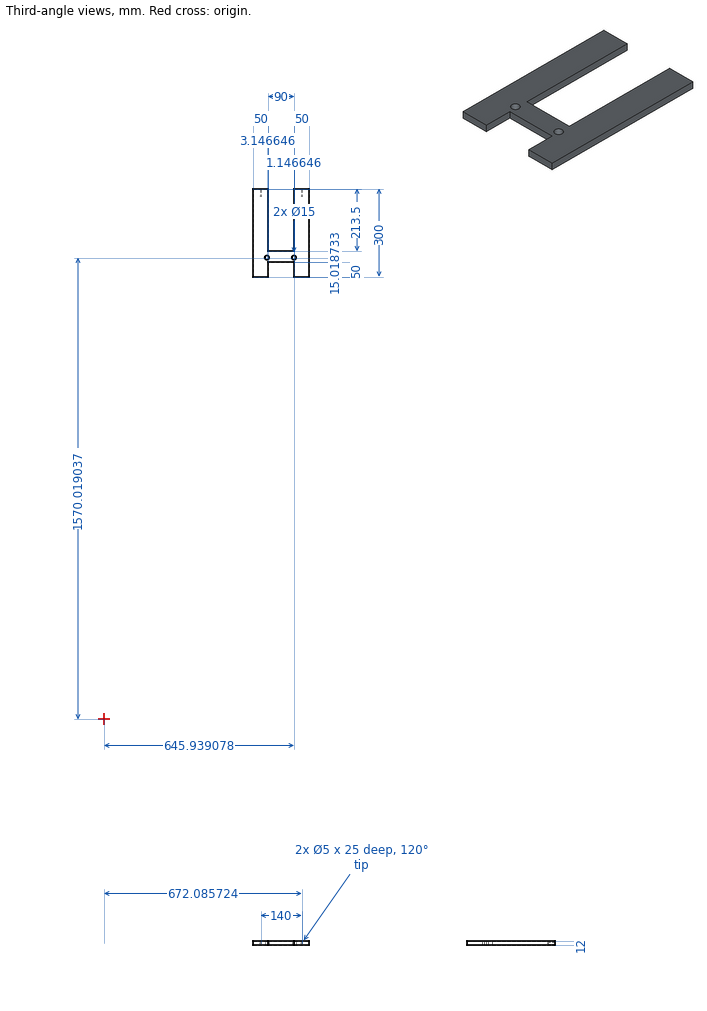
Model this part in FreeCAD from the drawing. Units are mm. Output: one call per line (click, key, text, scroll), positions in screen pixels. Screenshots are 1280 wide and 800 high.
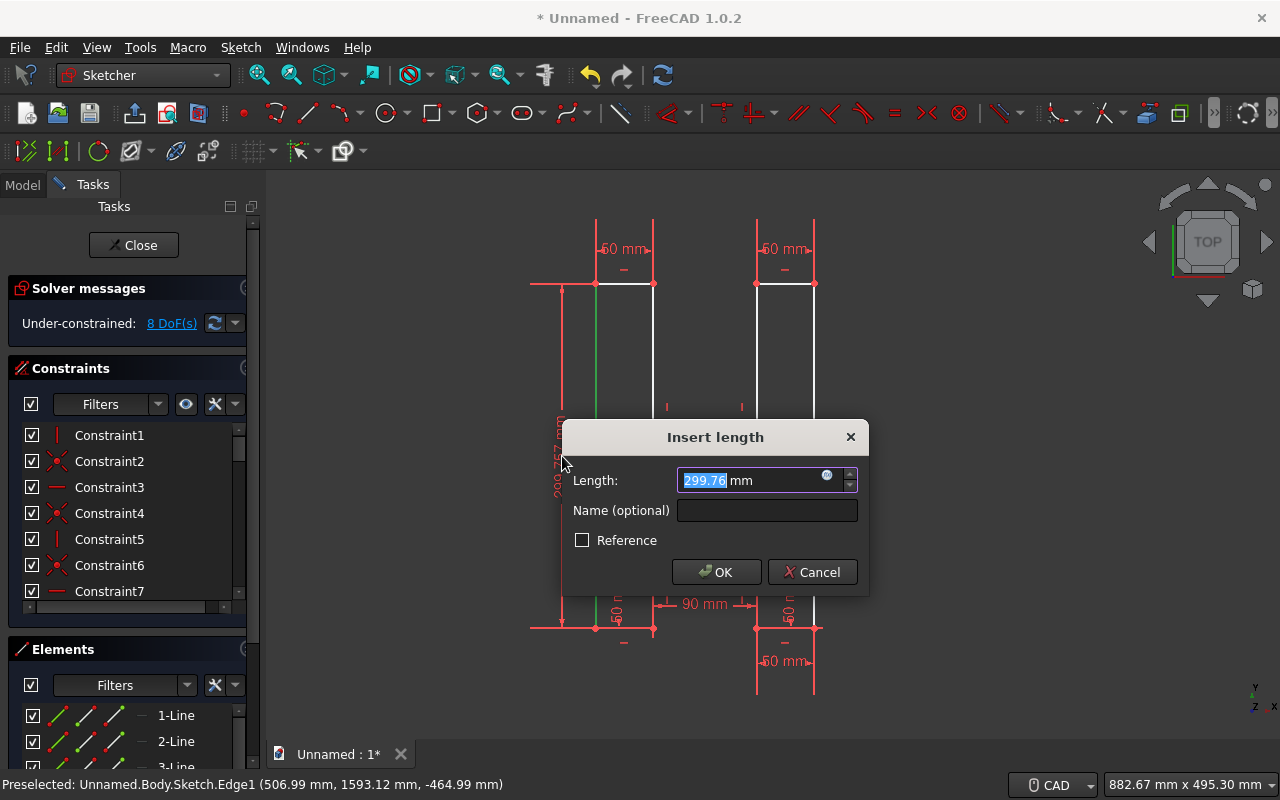
text(300)
key(Return)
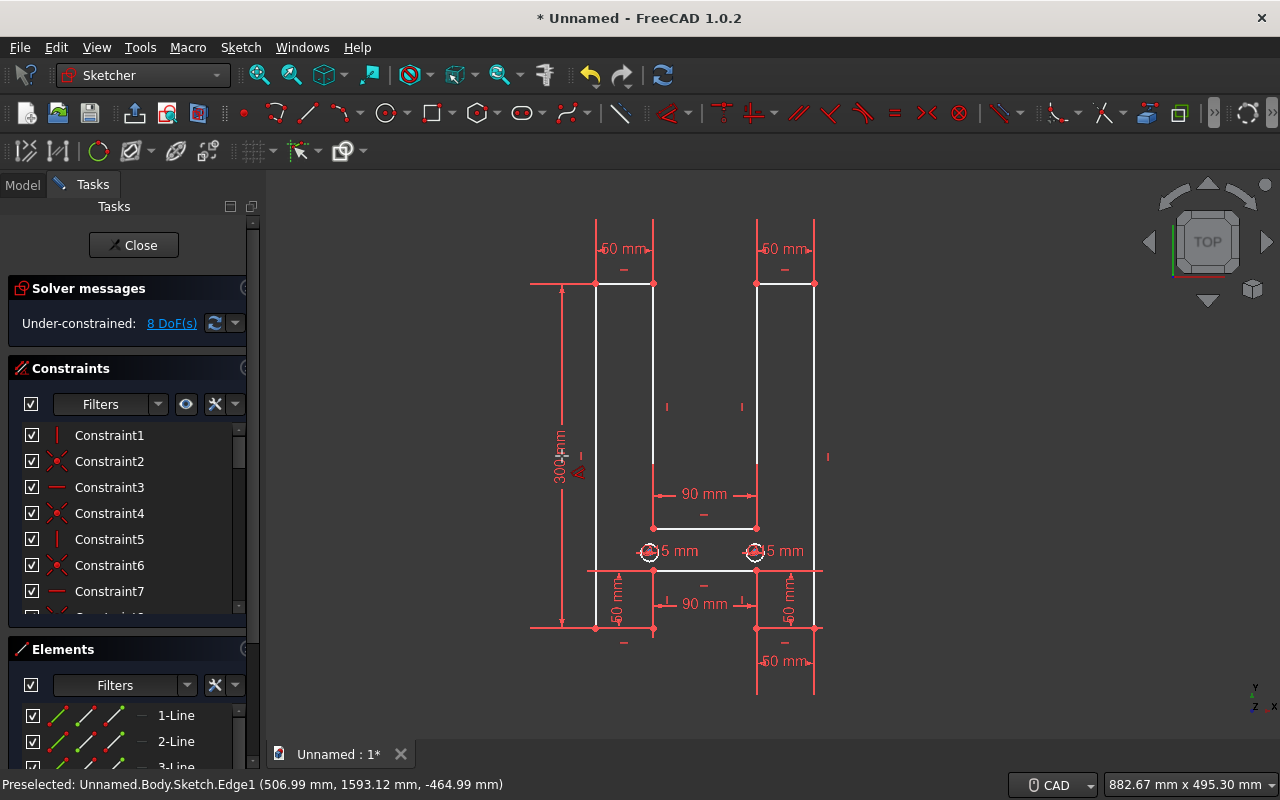
click(814, 387)
click(848, 456)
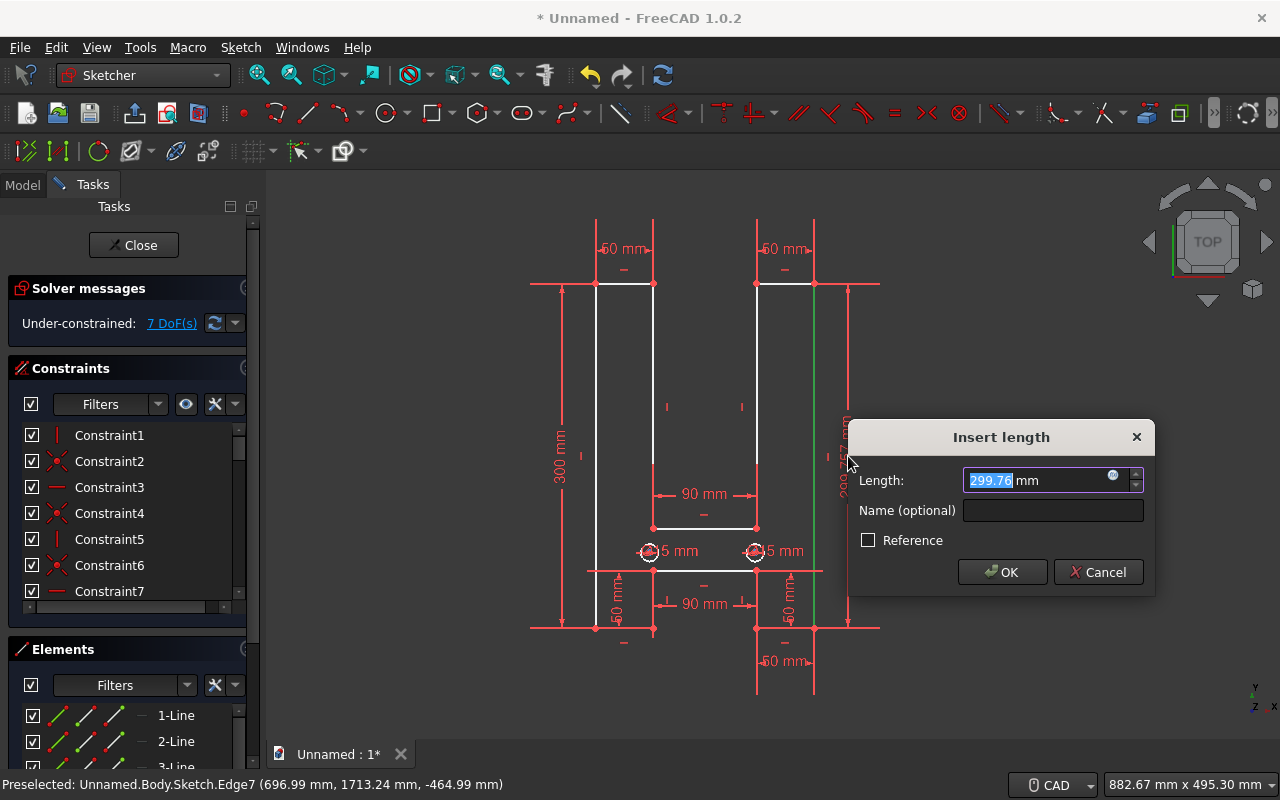
text(300)
key(Return)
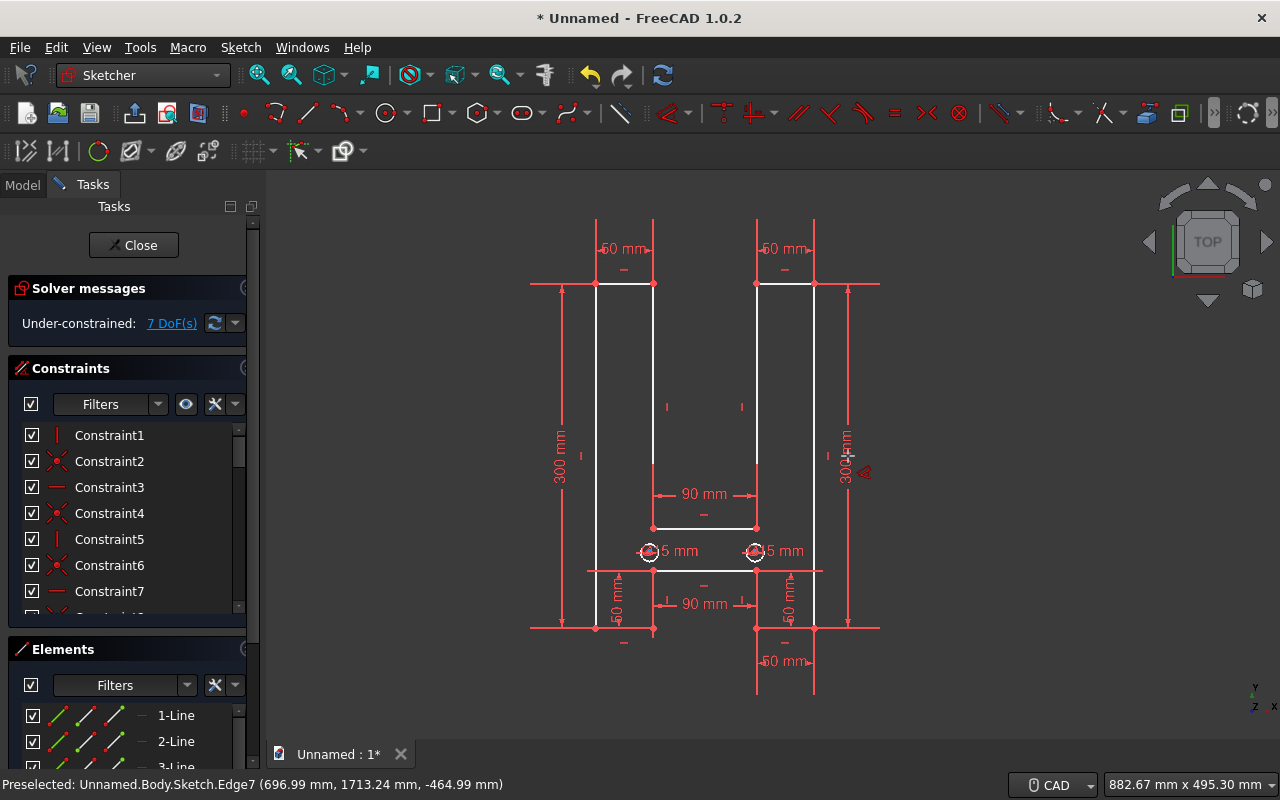
click(653, 357)
click(619, 406)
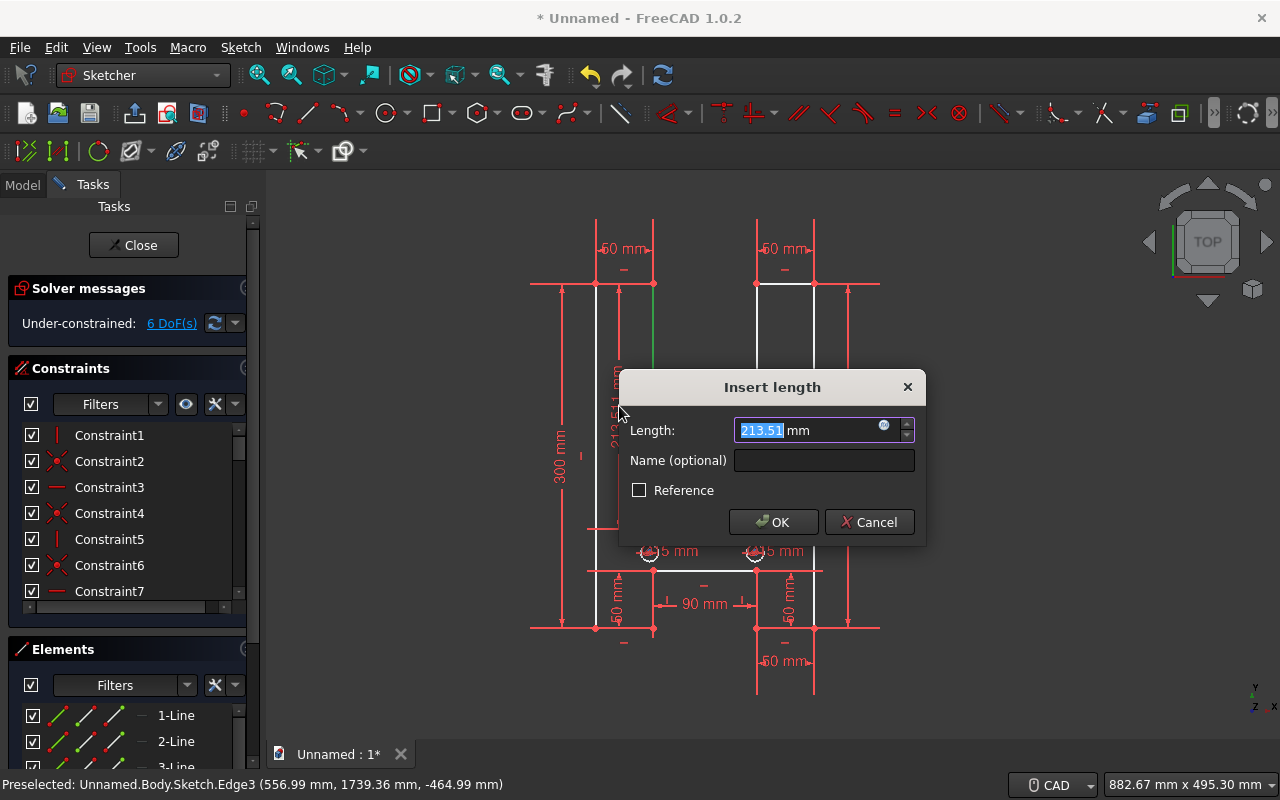
text(213.5)
key(Return)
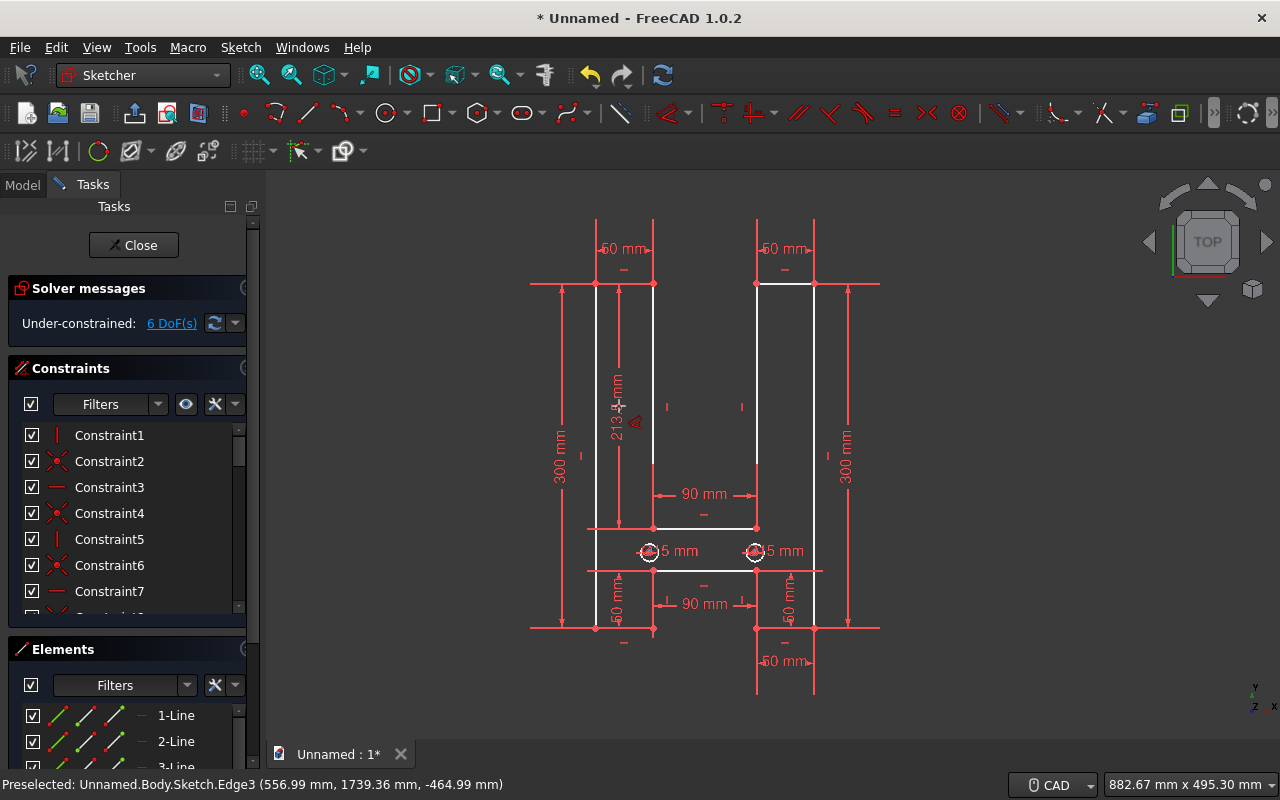
scroll(757, 571, up, 18)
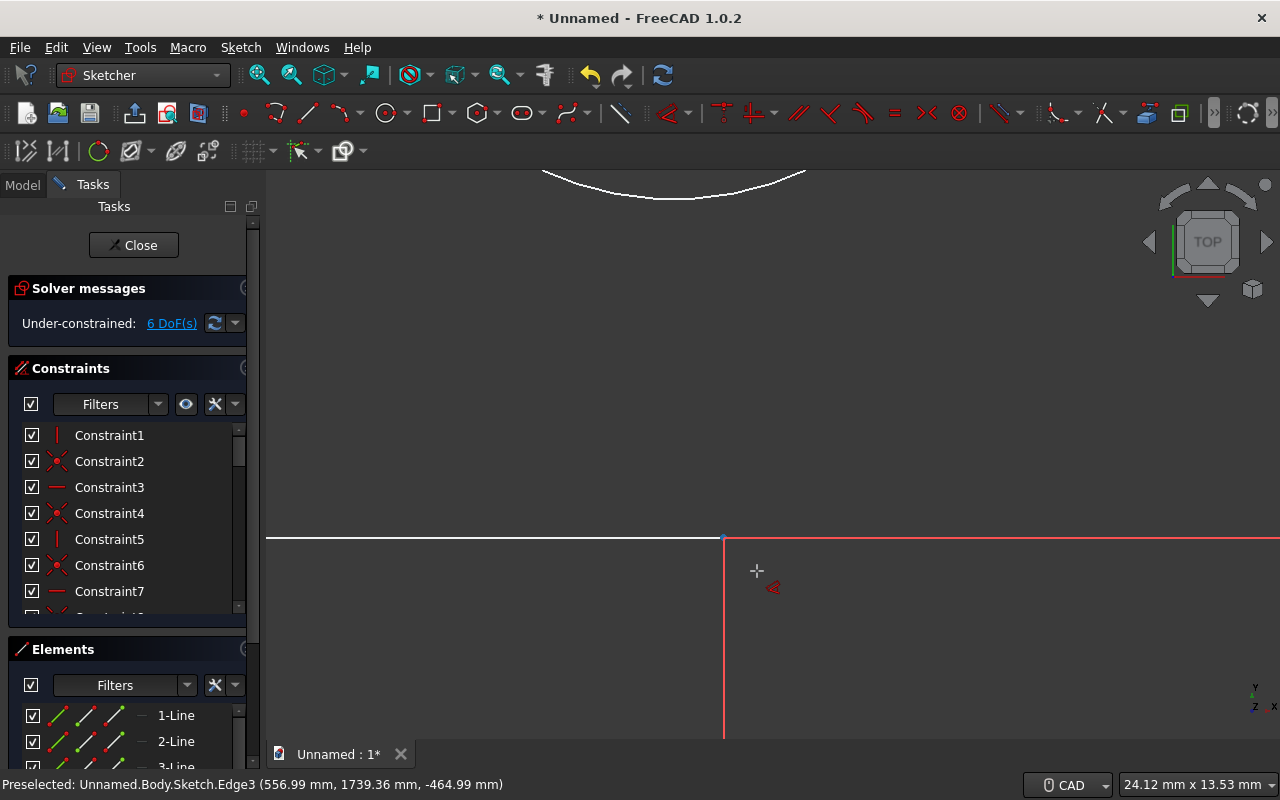
click(724, 538)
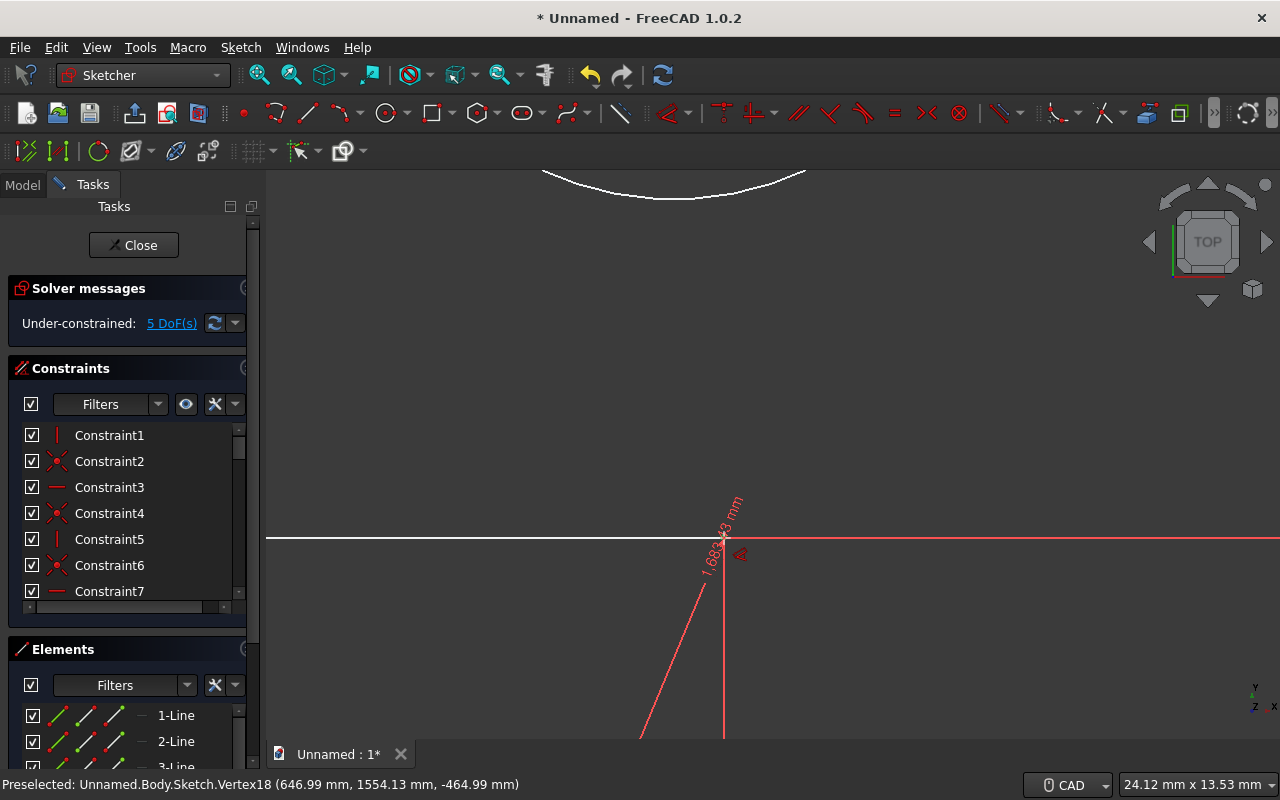
scroll(769, 598, down, 17)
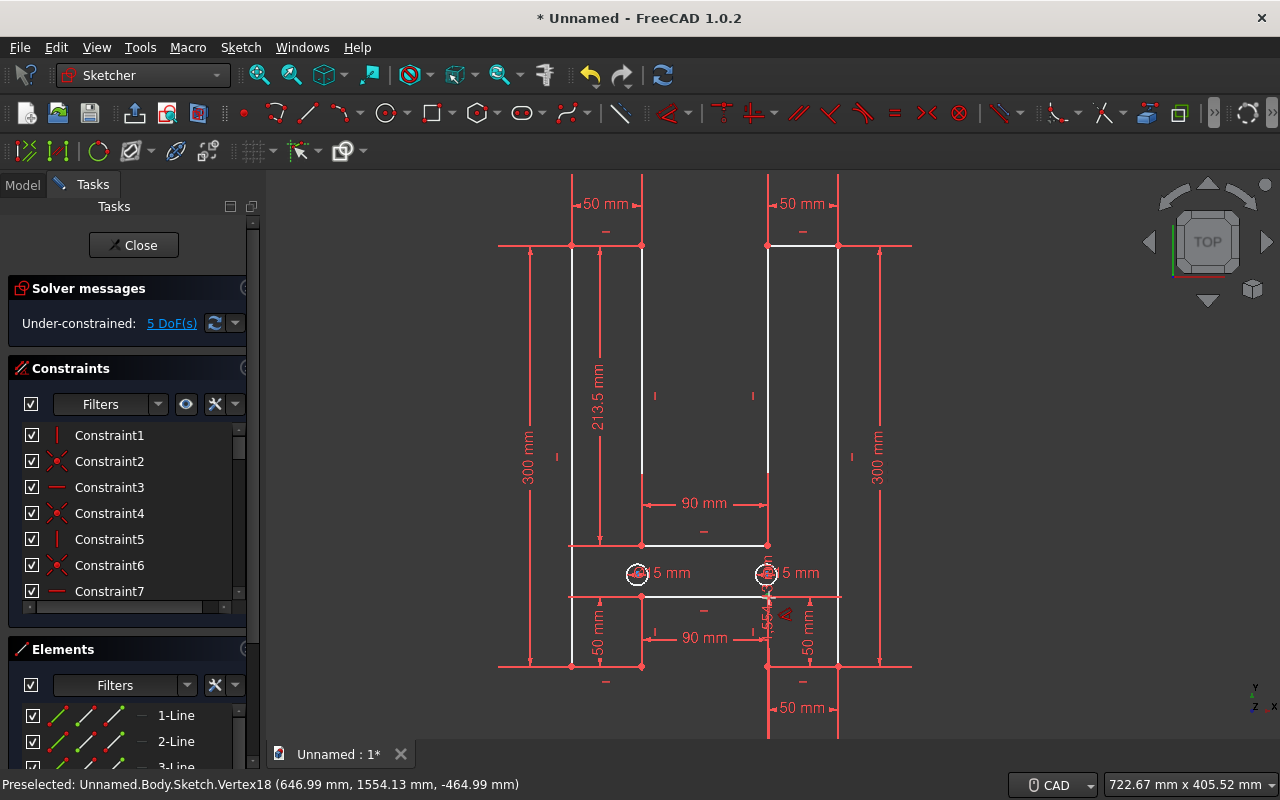
scroll(766, 575, up, 17)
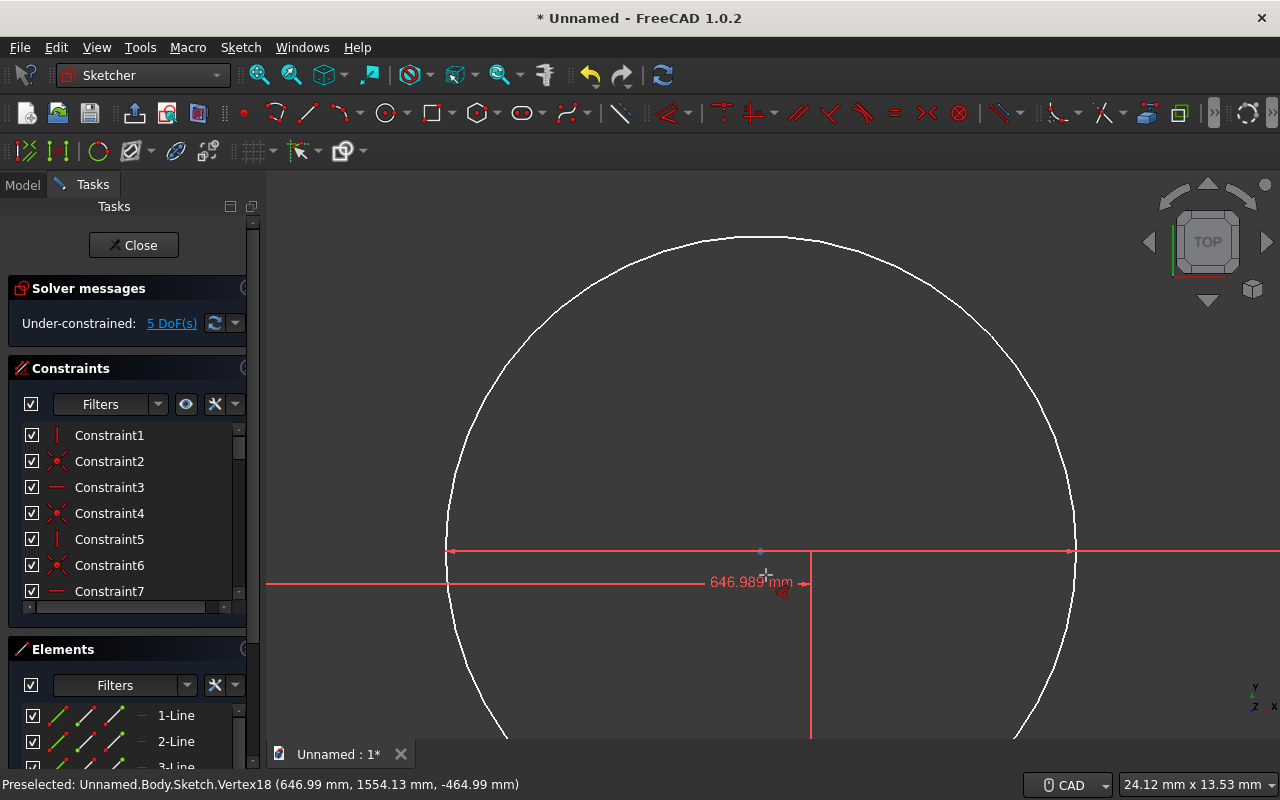
click(761, 551)
click(786, 517)